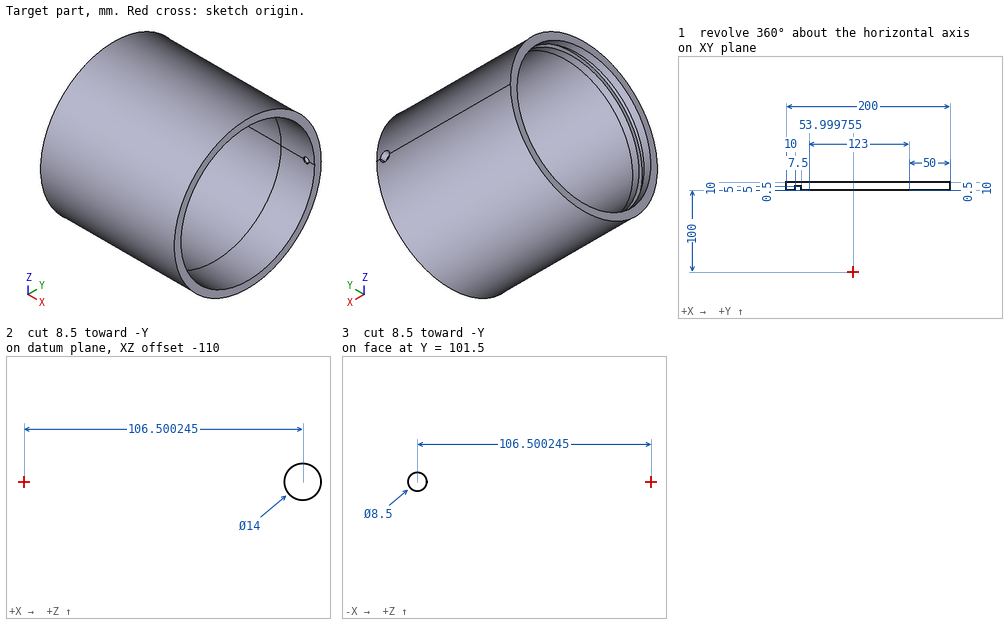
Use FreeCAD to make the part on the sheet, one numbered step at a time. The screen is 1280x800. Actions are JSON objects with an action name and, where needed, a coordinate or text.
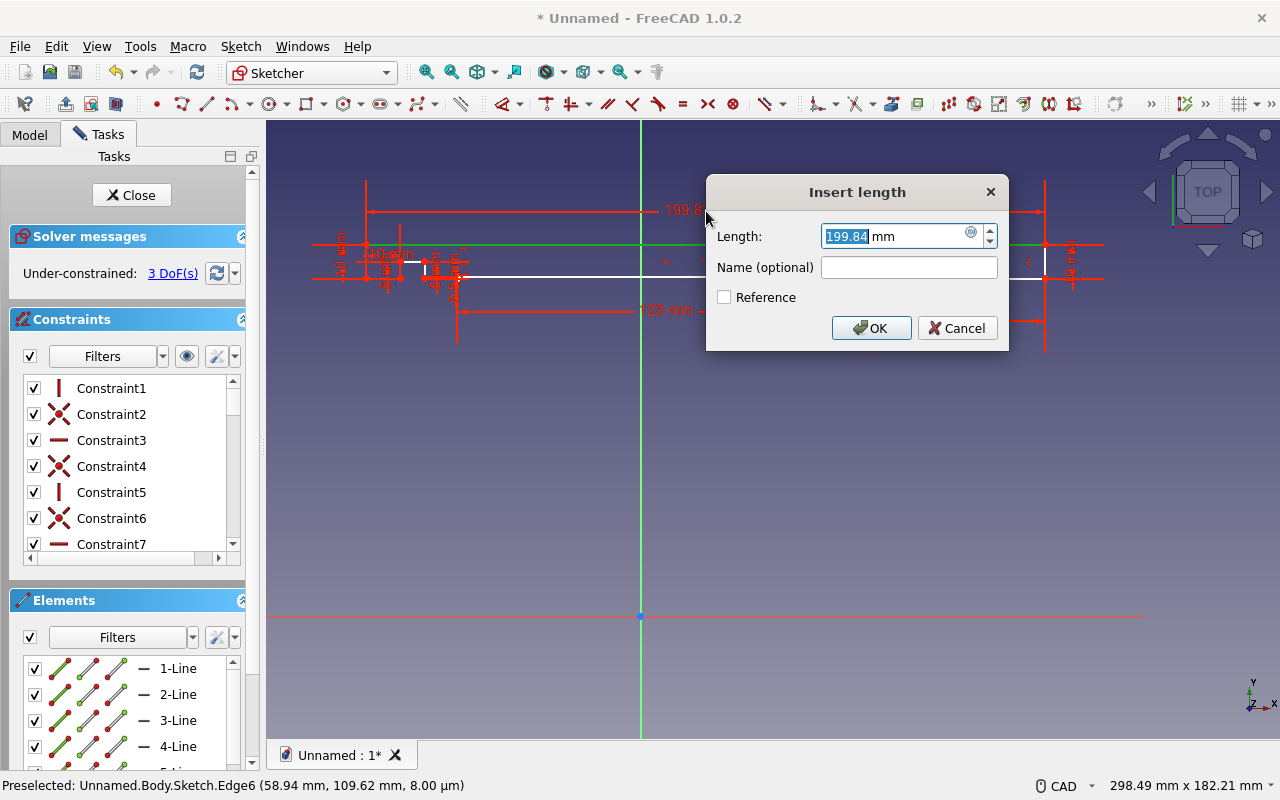
{"action": "type", "text": "200"}
{"action": "key", "text": "Return"}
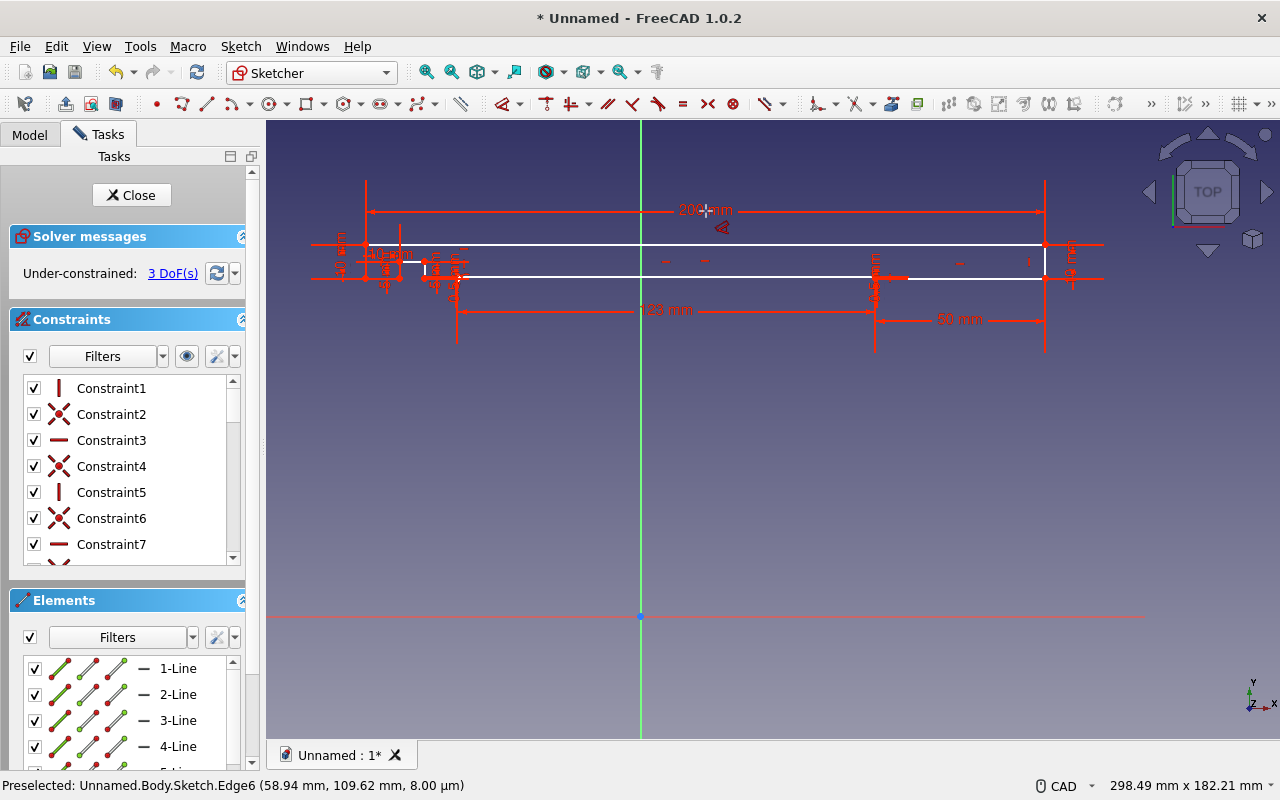
{"action": "scroll", "coordinate": [410, 262], "scroll_direction": "up", "scroll_amount": 3}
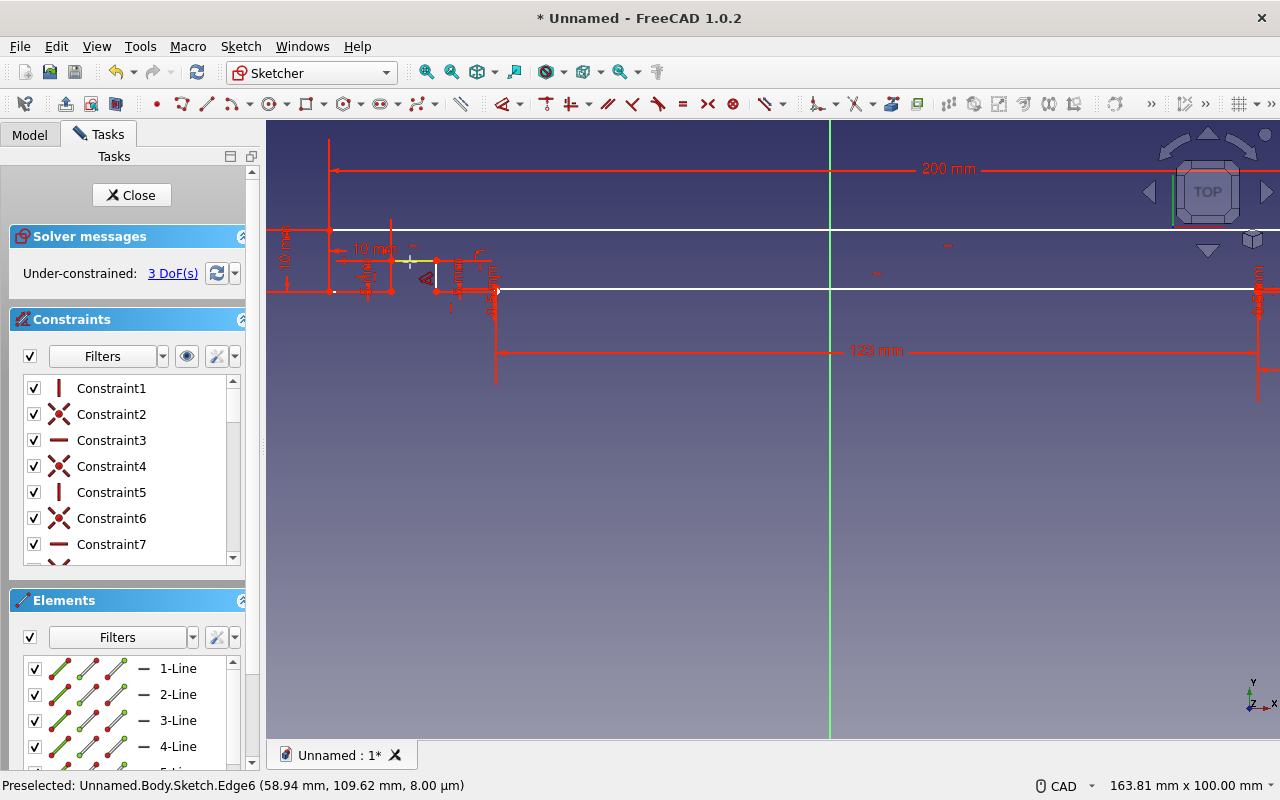
{"action": "left_click", "coordinate": [409, 261]}
{"action": "left_click", "coordinate": [414, 203]}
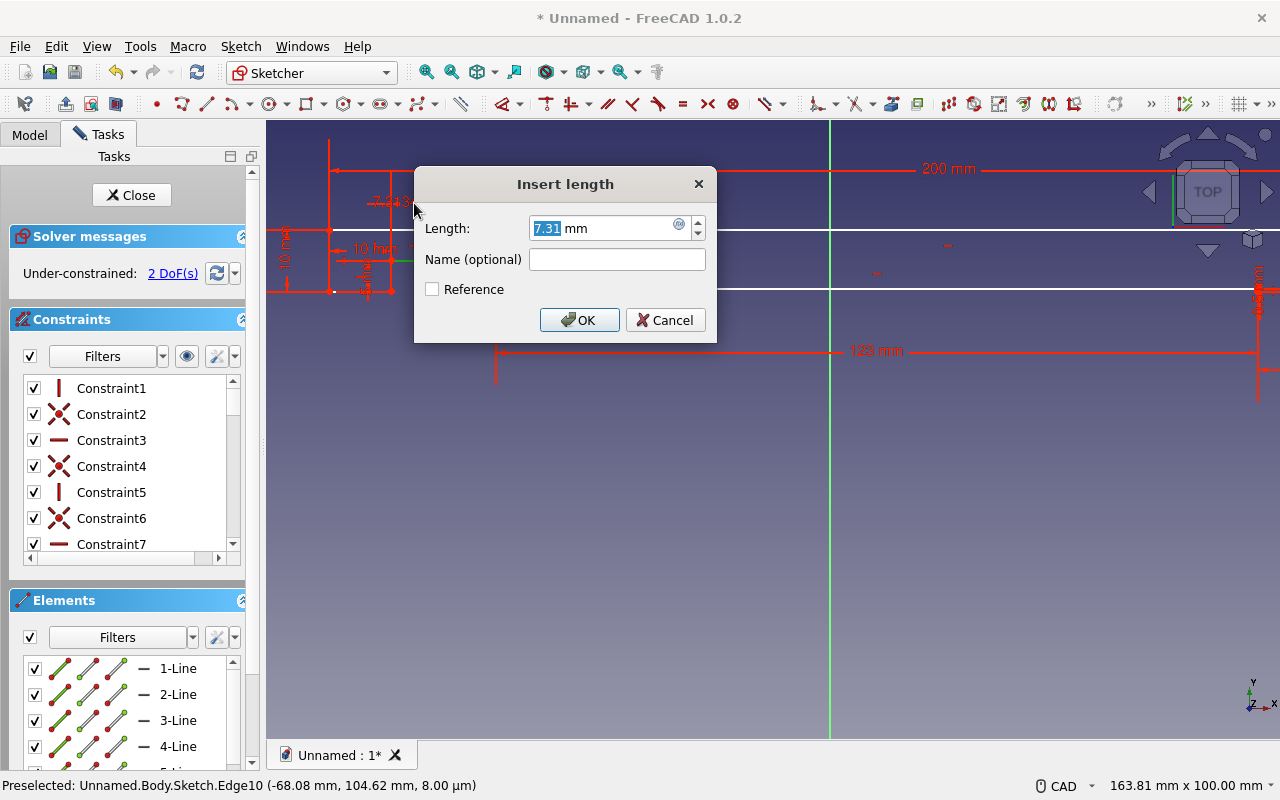
{"action": "type", "text": "7.5"}
{"action": "key", "text": "Return"}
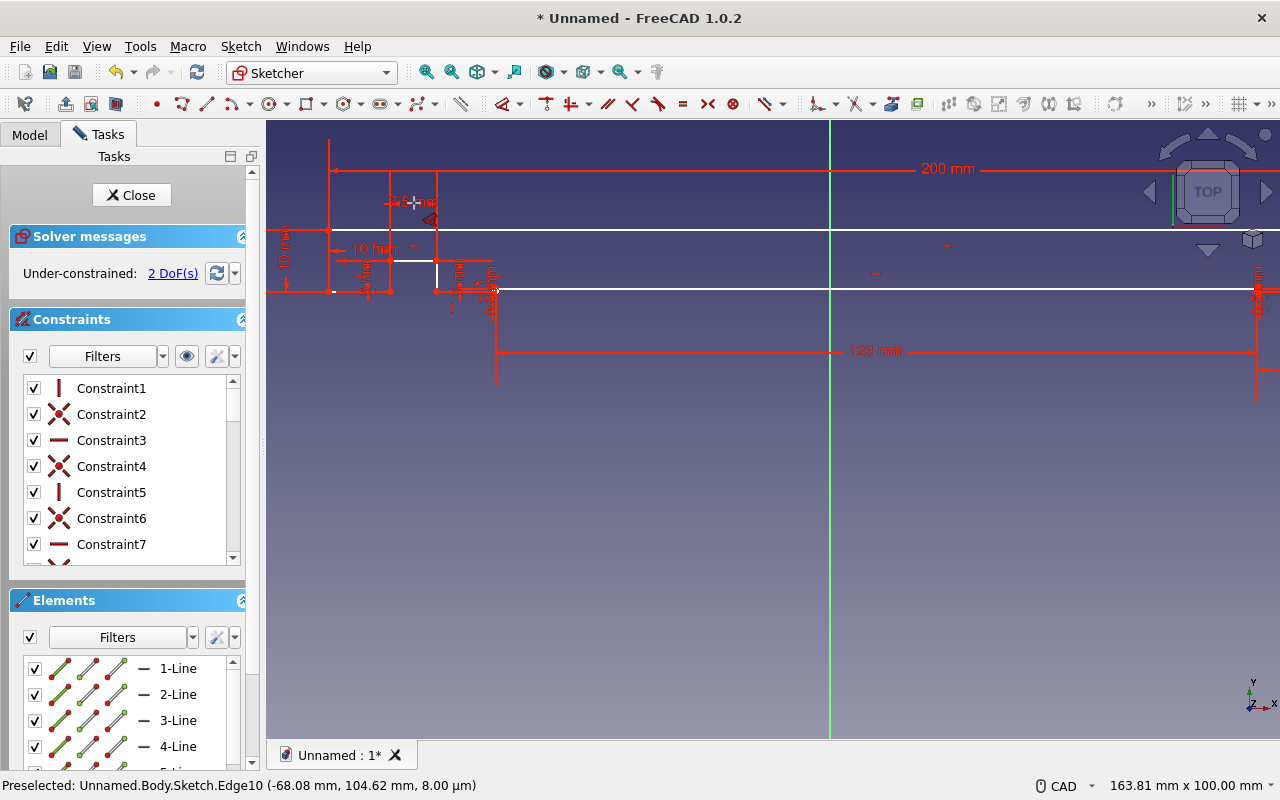
{"action": "scroll", "coordinate": [496, 292], "scroll_direction": "up", "scroll_amount": 7}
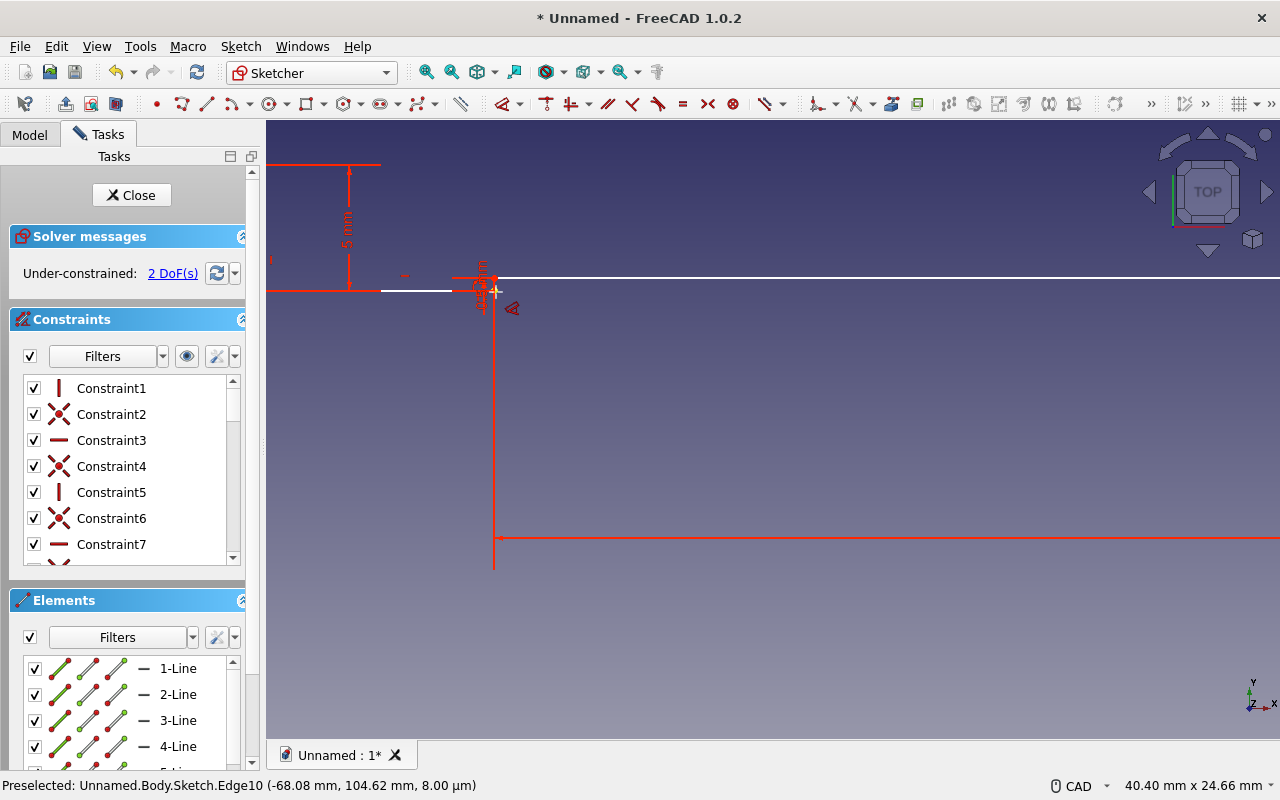
{"action": "left_click", "coordinate": [494, 291]}
{"action": "left_click", "coordinate": [460, 501]}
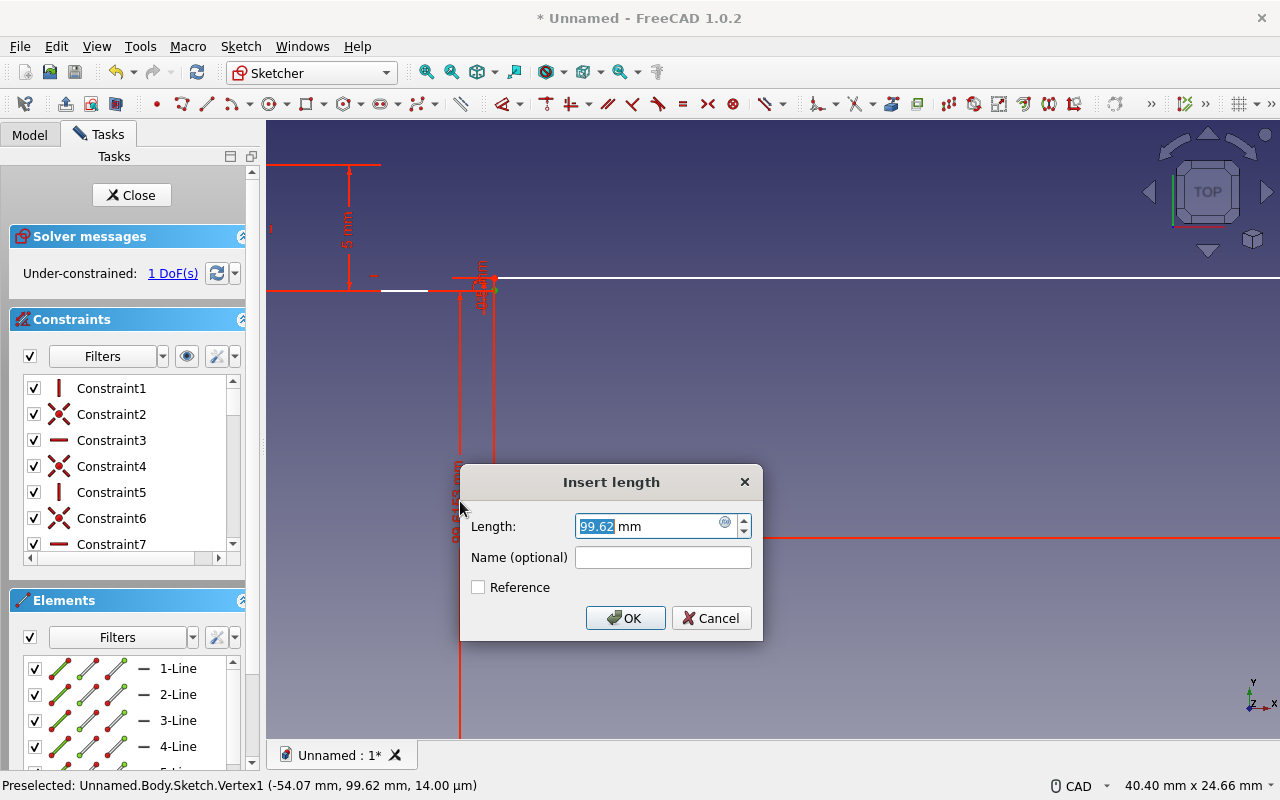
{"action": "type", "text": "100"}
{"action": "key", "text": "Return"}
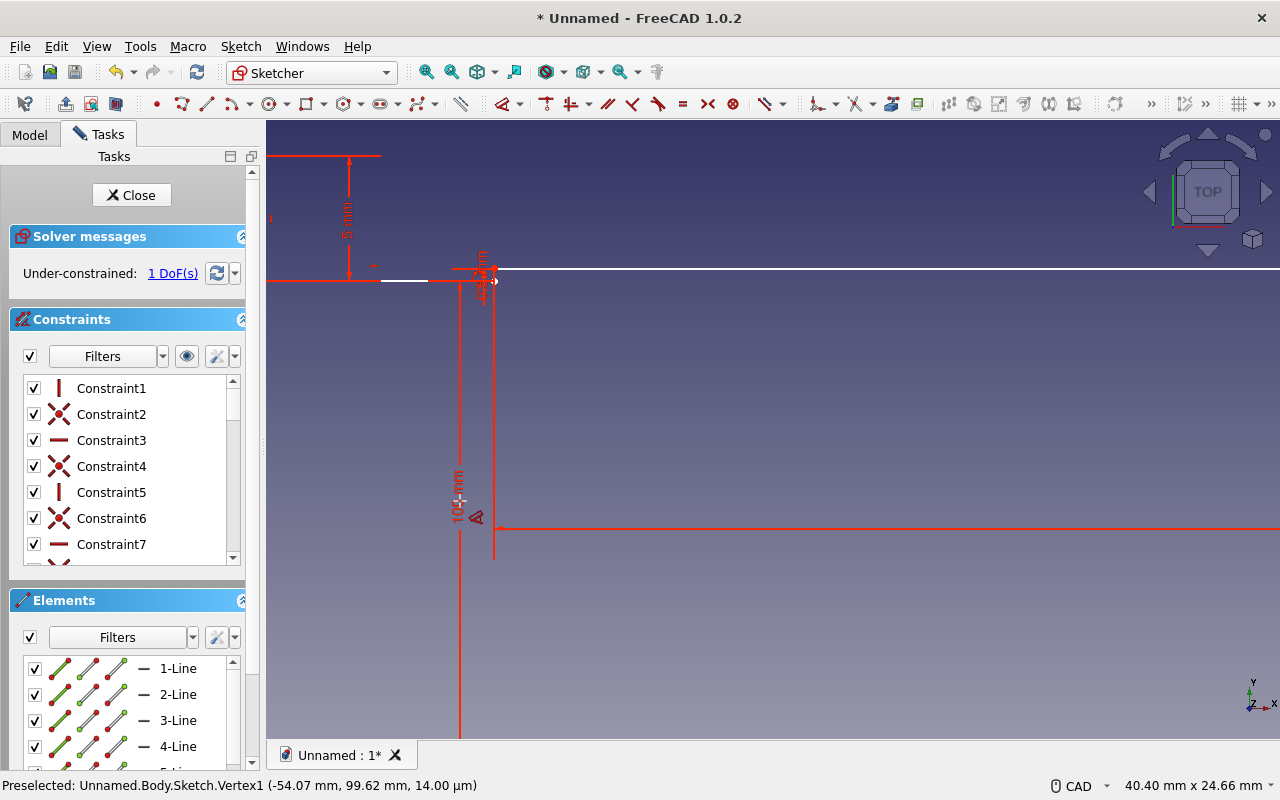
{"action": "left_click", "coordinate": [494, 281]}
{"action": "left_click", "coordinate": [805, 247]}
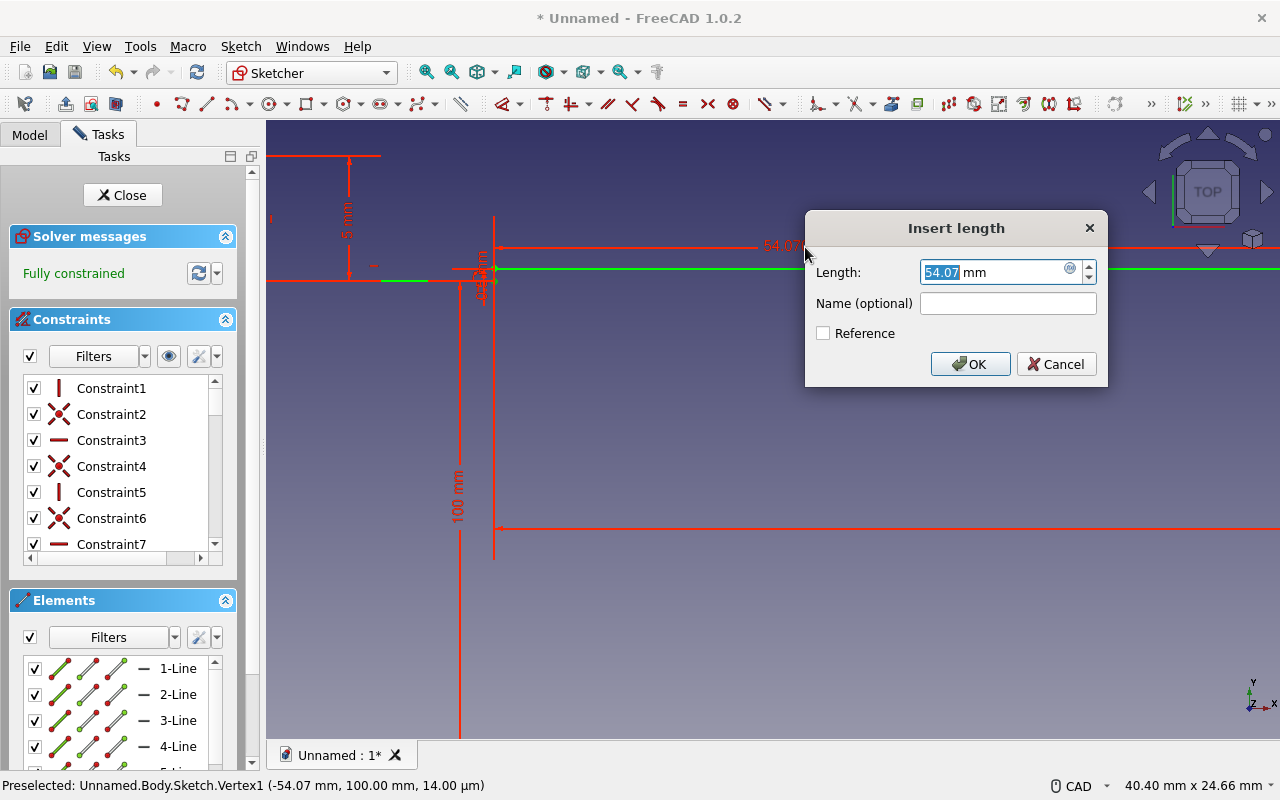
{"action": "type", "text": "53.999755"}
{"action": "key", "text": "Return"}
{"action": "key", "text": "Escape"}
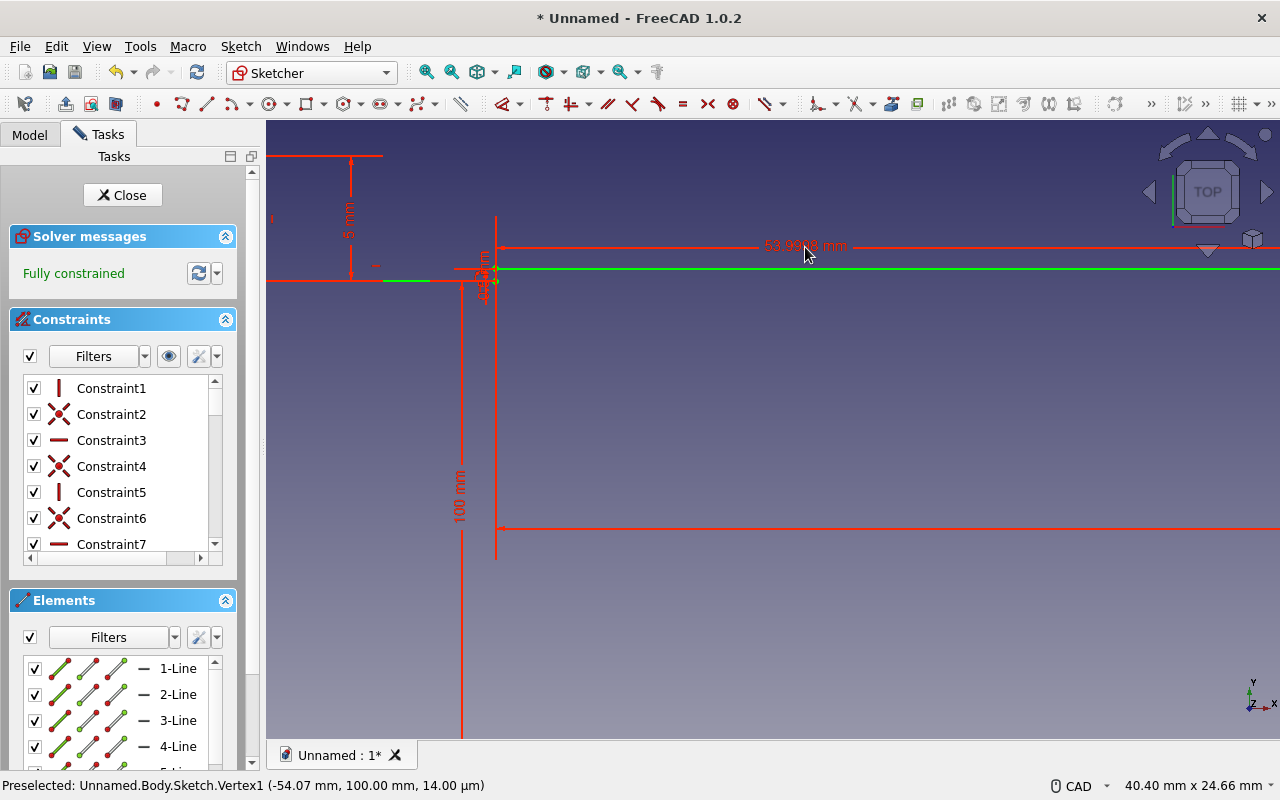
{"action": "left_click", "coordinate": [123, 195]}